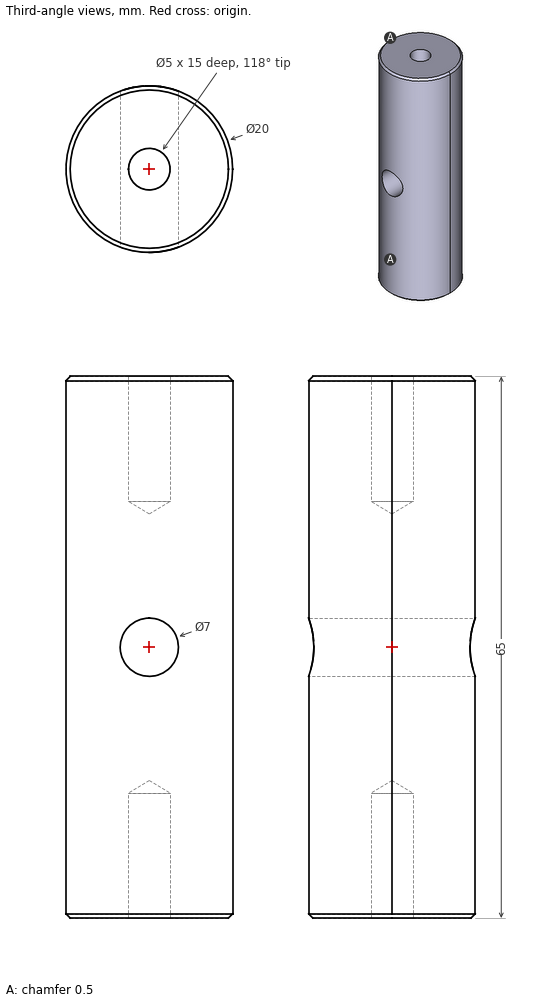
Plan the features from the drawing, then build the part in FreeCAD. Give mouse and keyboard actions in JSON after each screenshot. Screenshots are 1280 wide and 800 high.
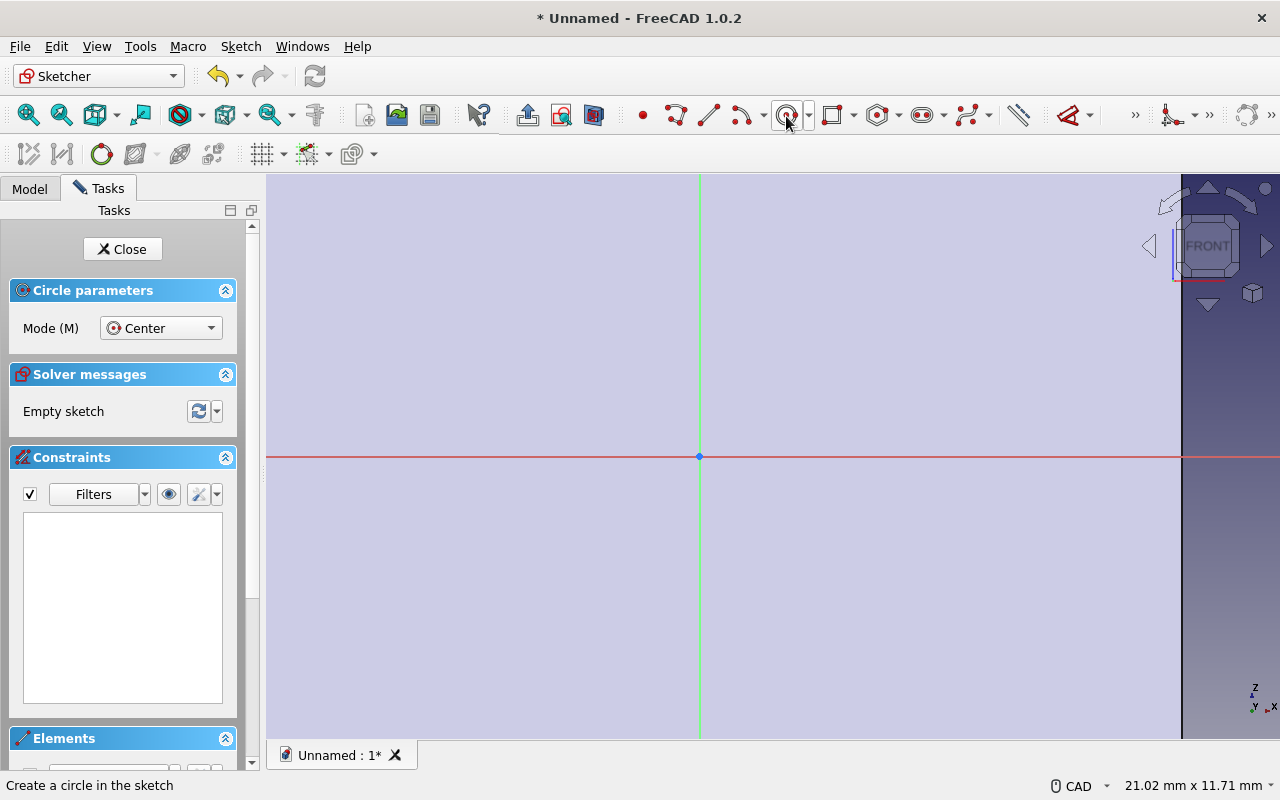
{"action": "left_click", "coordinate": [700, 456]}
{"action": "left_click", "coordinate": [819, 337]}
{"action": "key", "text": "Escape"}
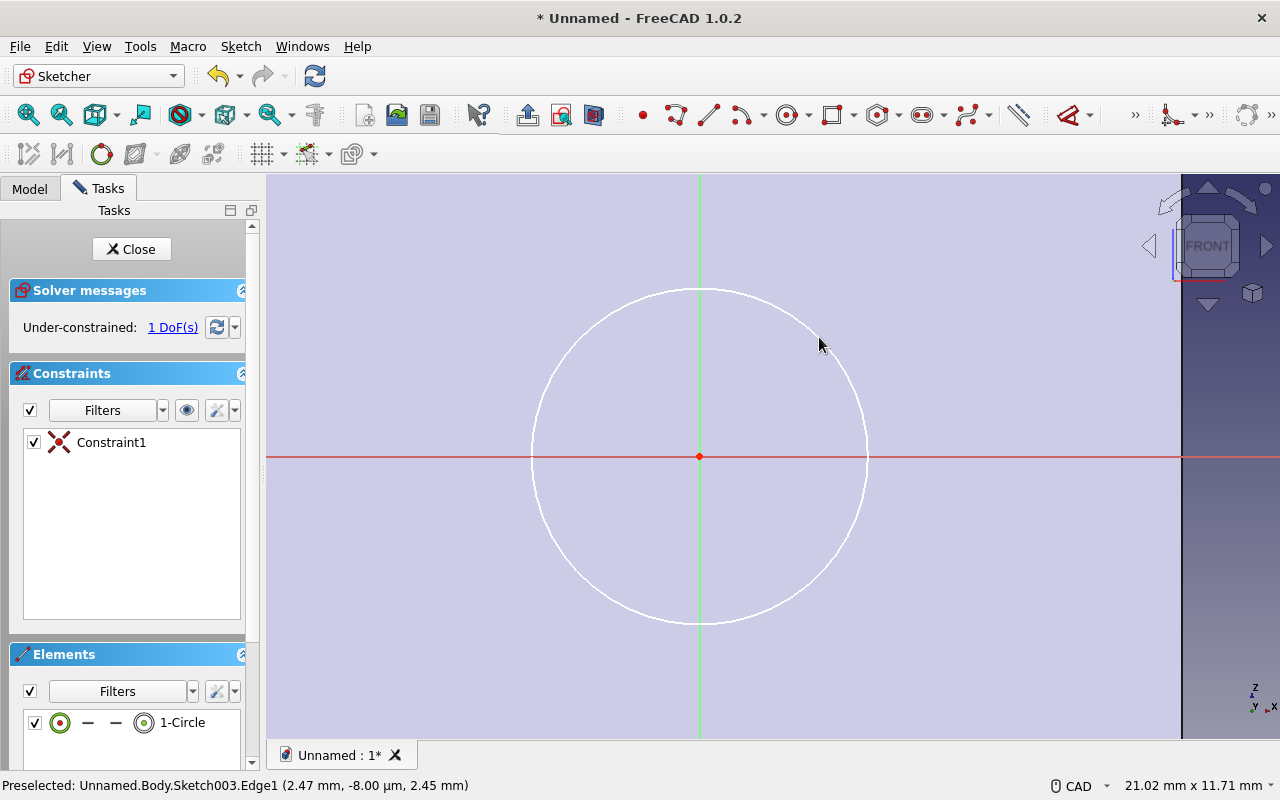
{"action": "left_click", "coordinate": [1068, 116]}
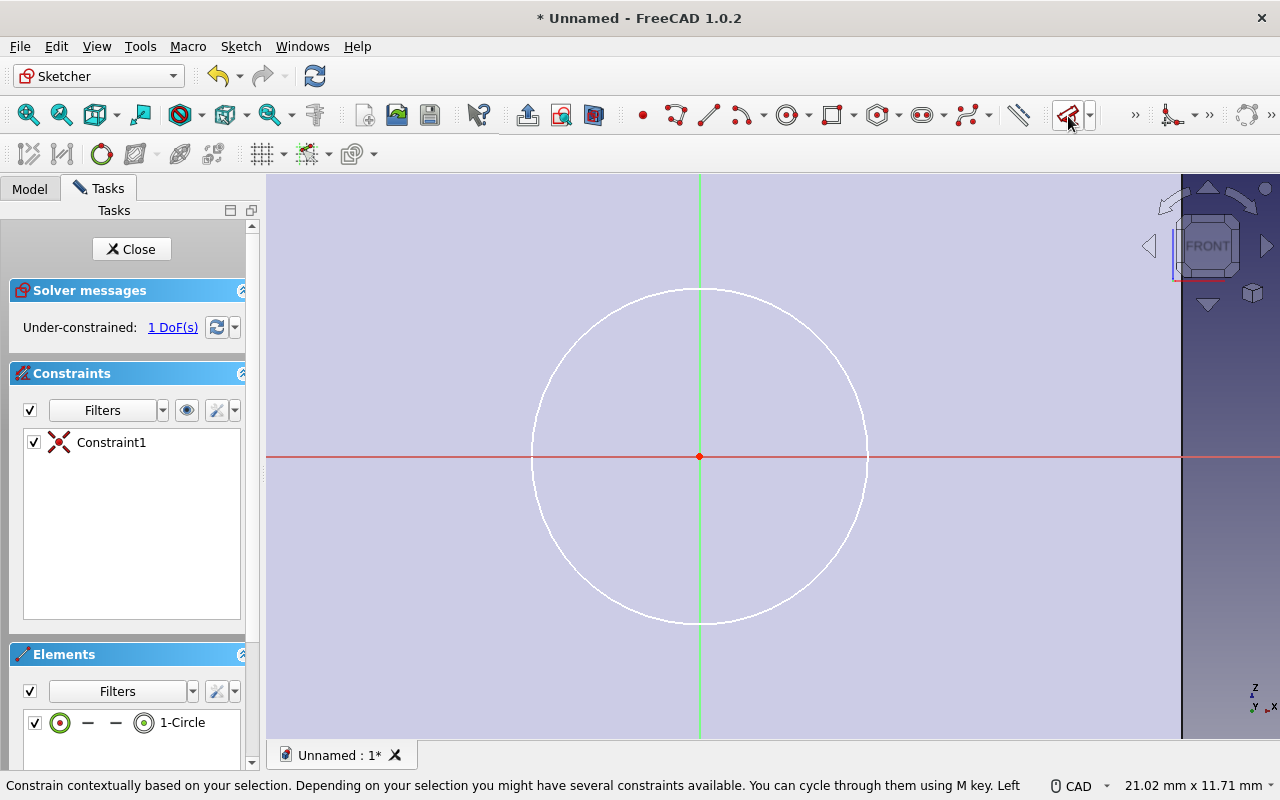
{"action": "left_click", "coordinate": [818, 337]}
{"action": "left_click", "coordinate": [841, 314]}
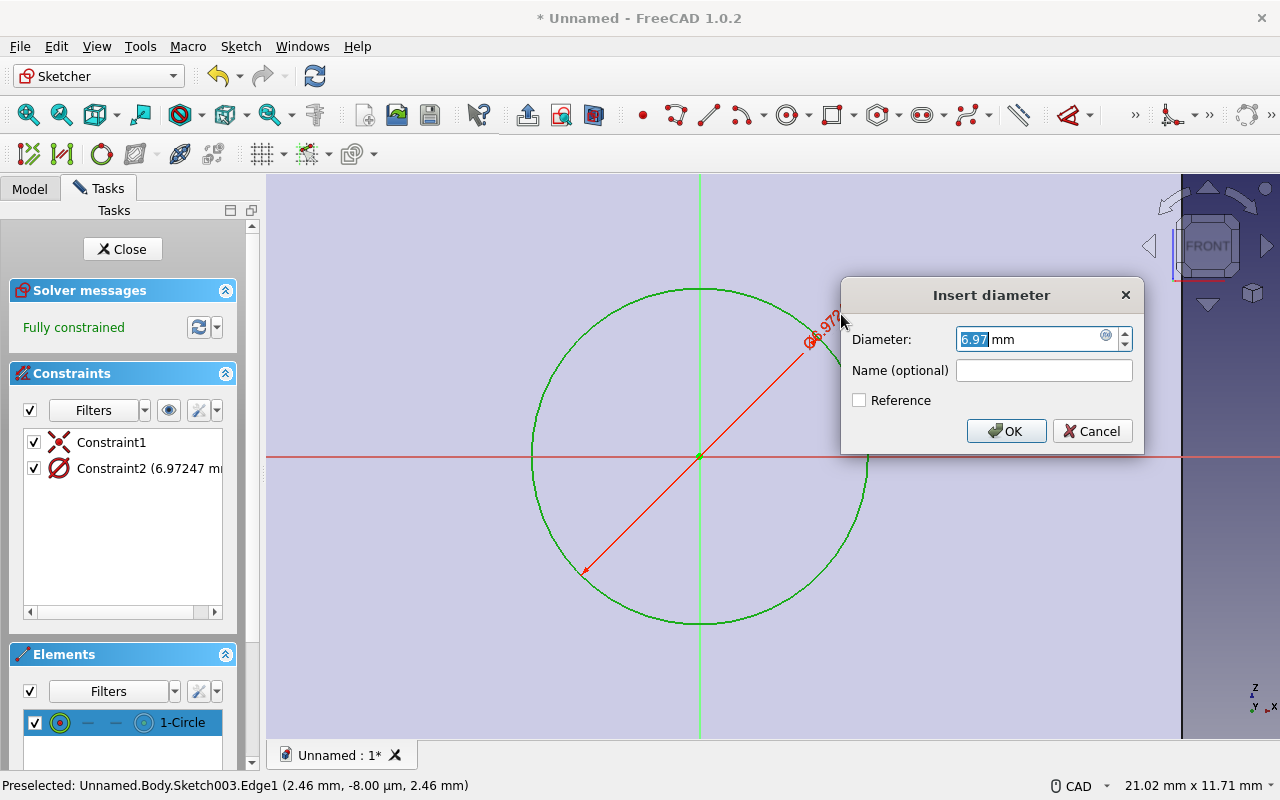
{"action": "type", "text": "7"}
{"action": "key", "text": "Return"}
{"action": "key", "text": "Escape"}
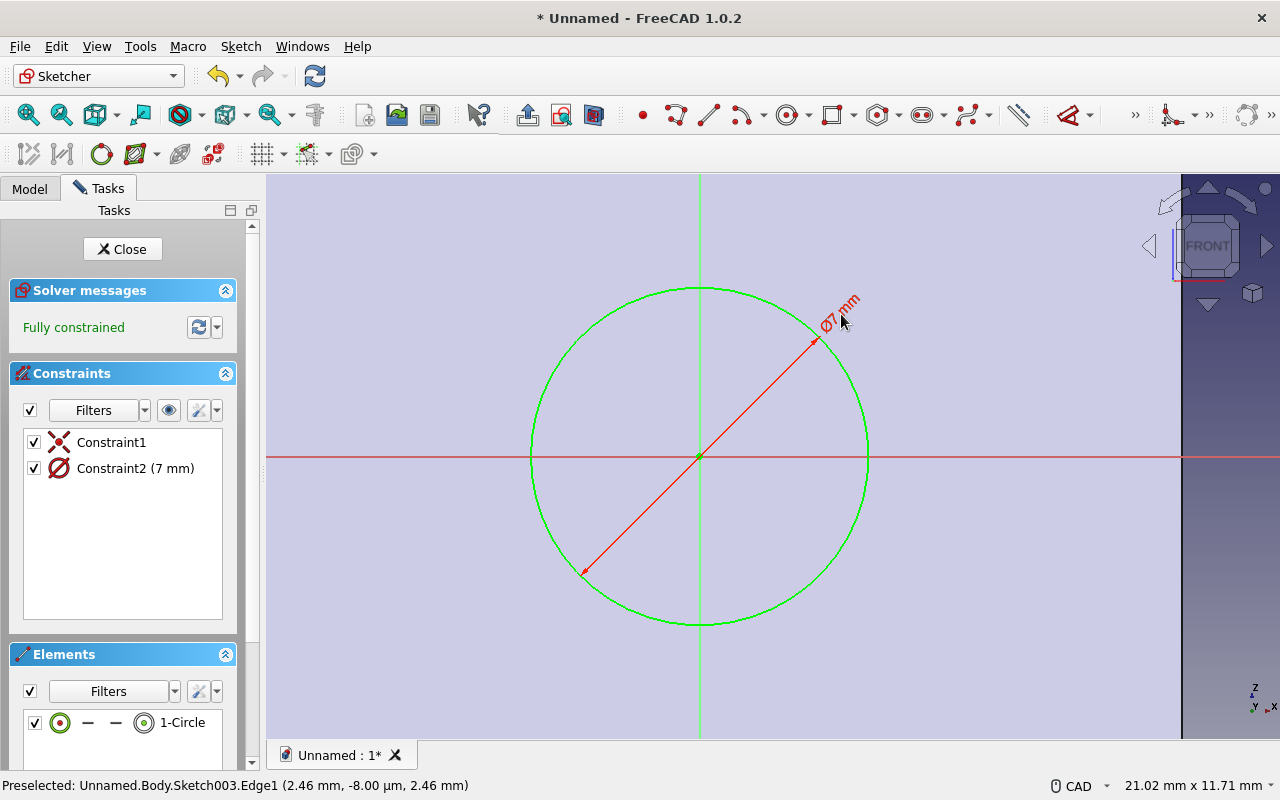
{"action": "left_click", "coordinate": [123, 249]}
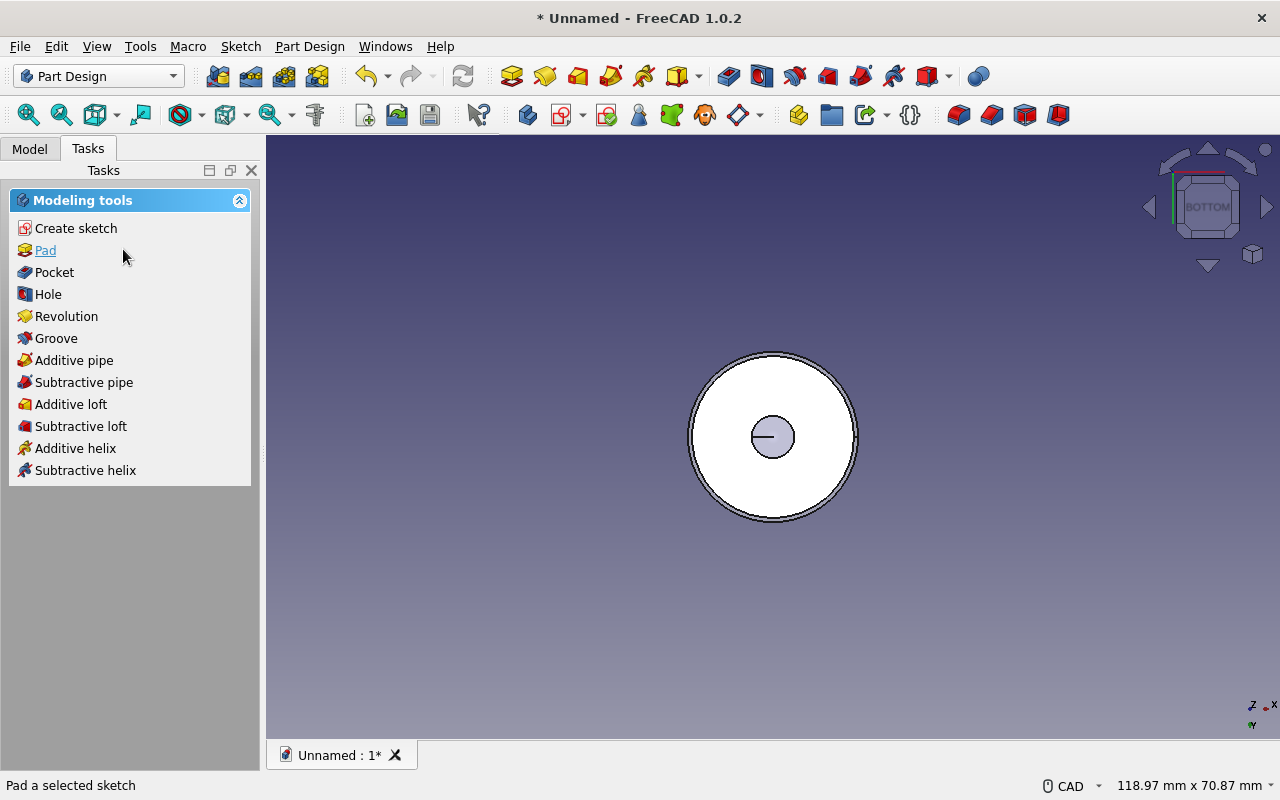
{"action": "left_click", "coordinate": [729, 76]}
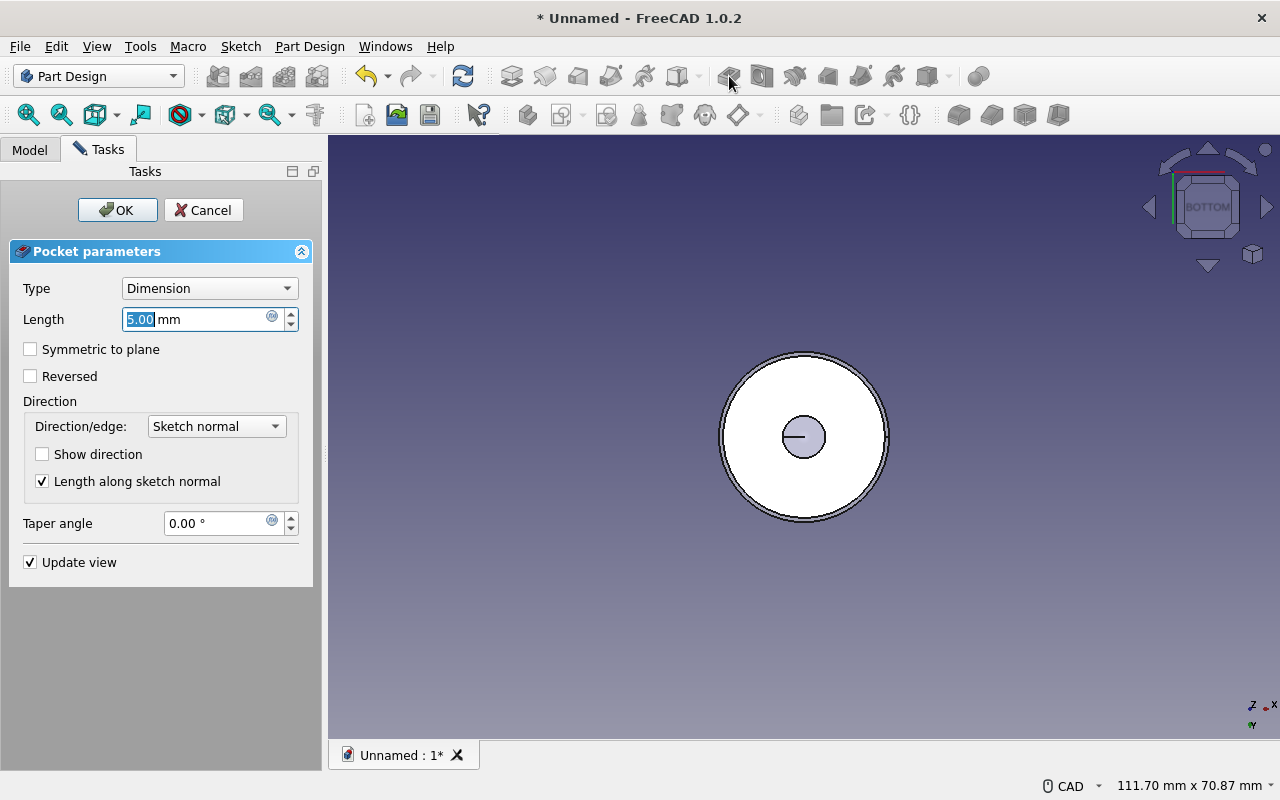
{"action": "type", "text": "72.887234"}
{"action": "key", "text": "Tab"}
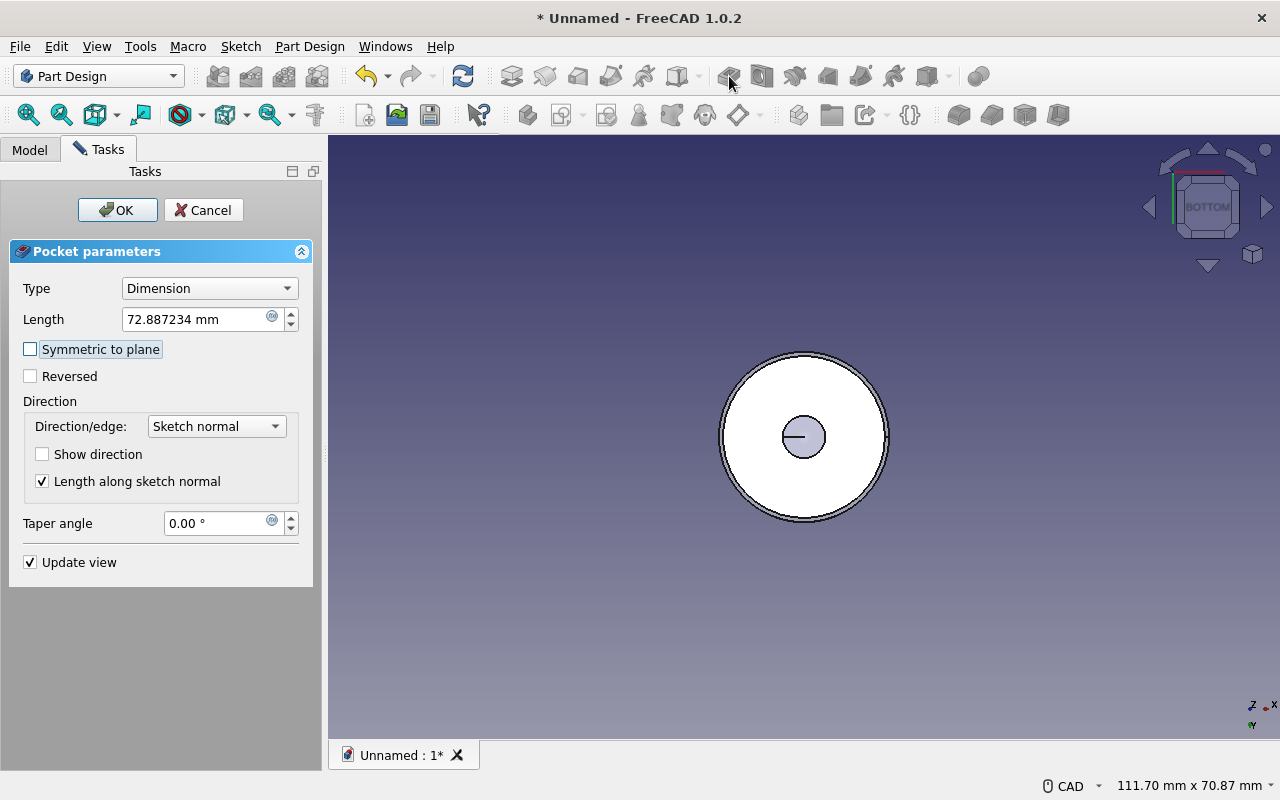
{"action": "left_click", "coordinate": [31, 349]}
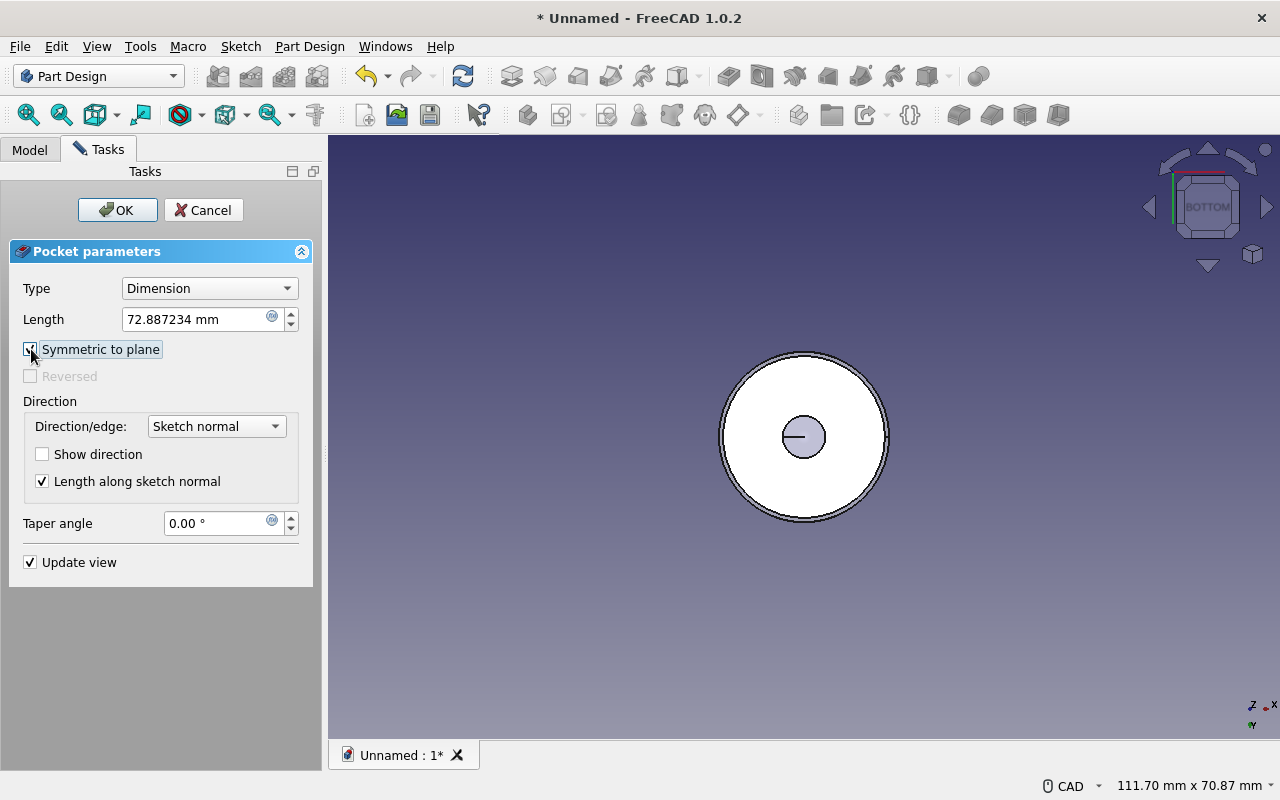
{"action": "left_click", "coordinate": [118, 210]}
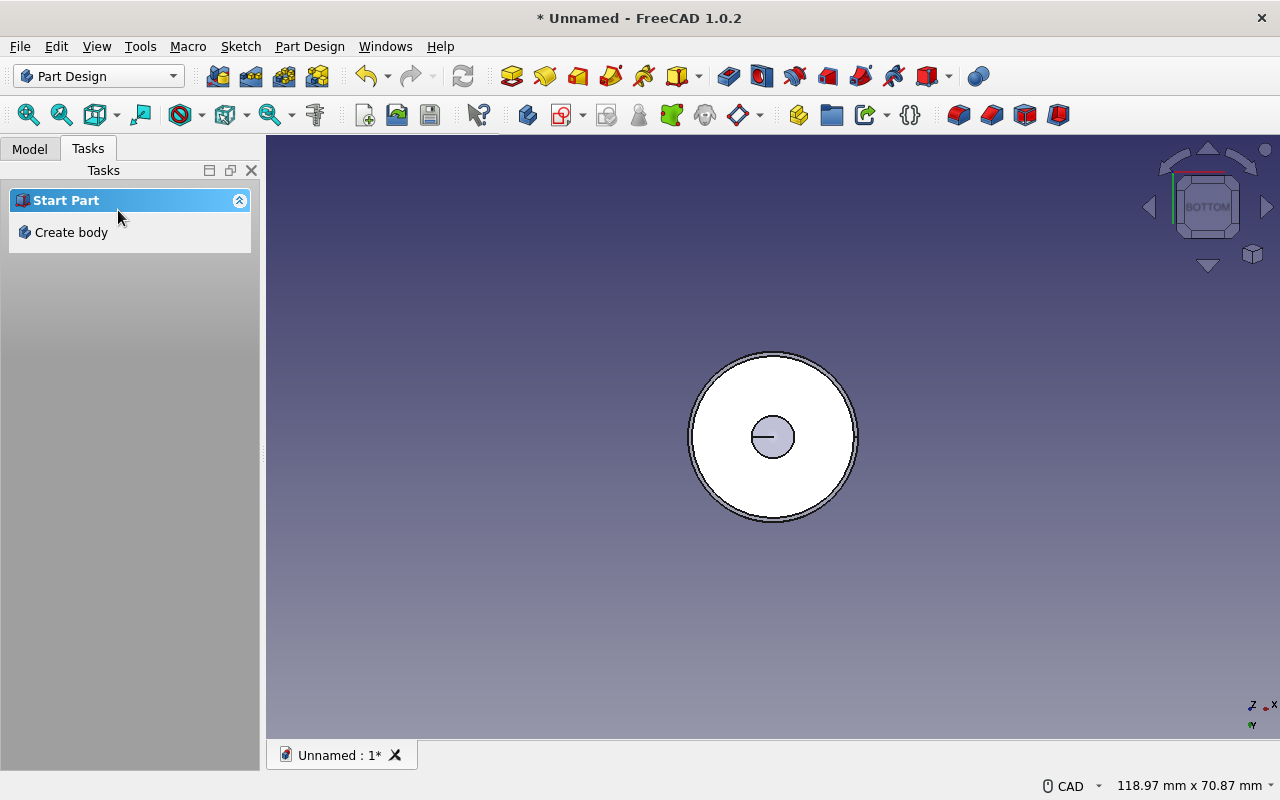
{"action": "key", "text": "0"}